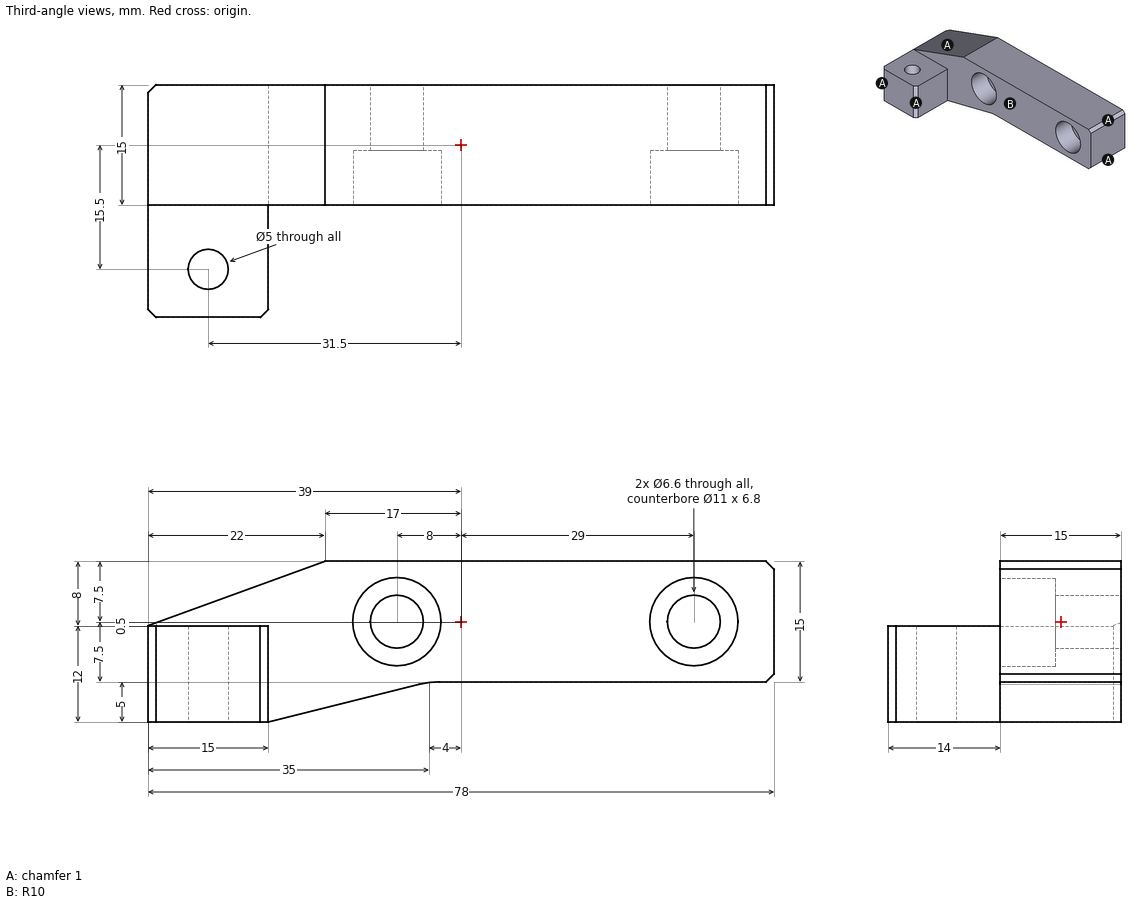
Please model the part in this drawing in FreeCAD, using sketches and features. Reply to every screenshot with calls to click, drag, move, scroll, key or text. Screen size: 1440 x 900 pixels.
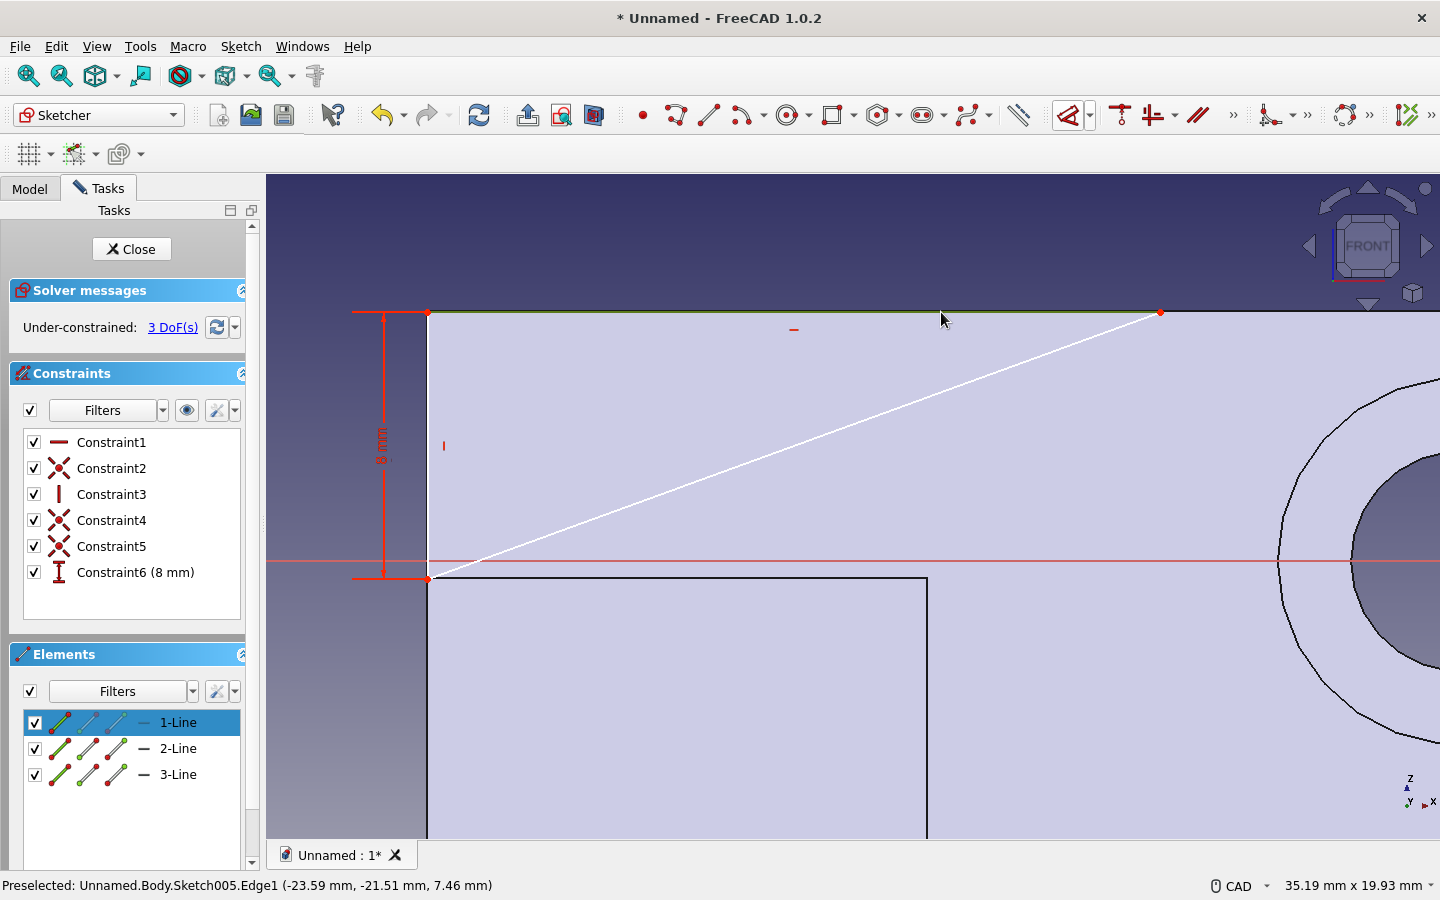
key(l)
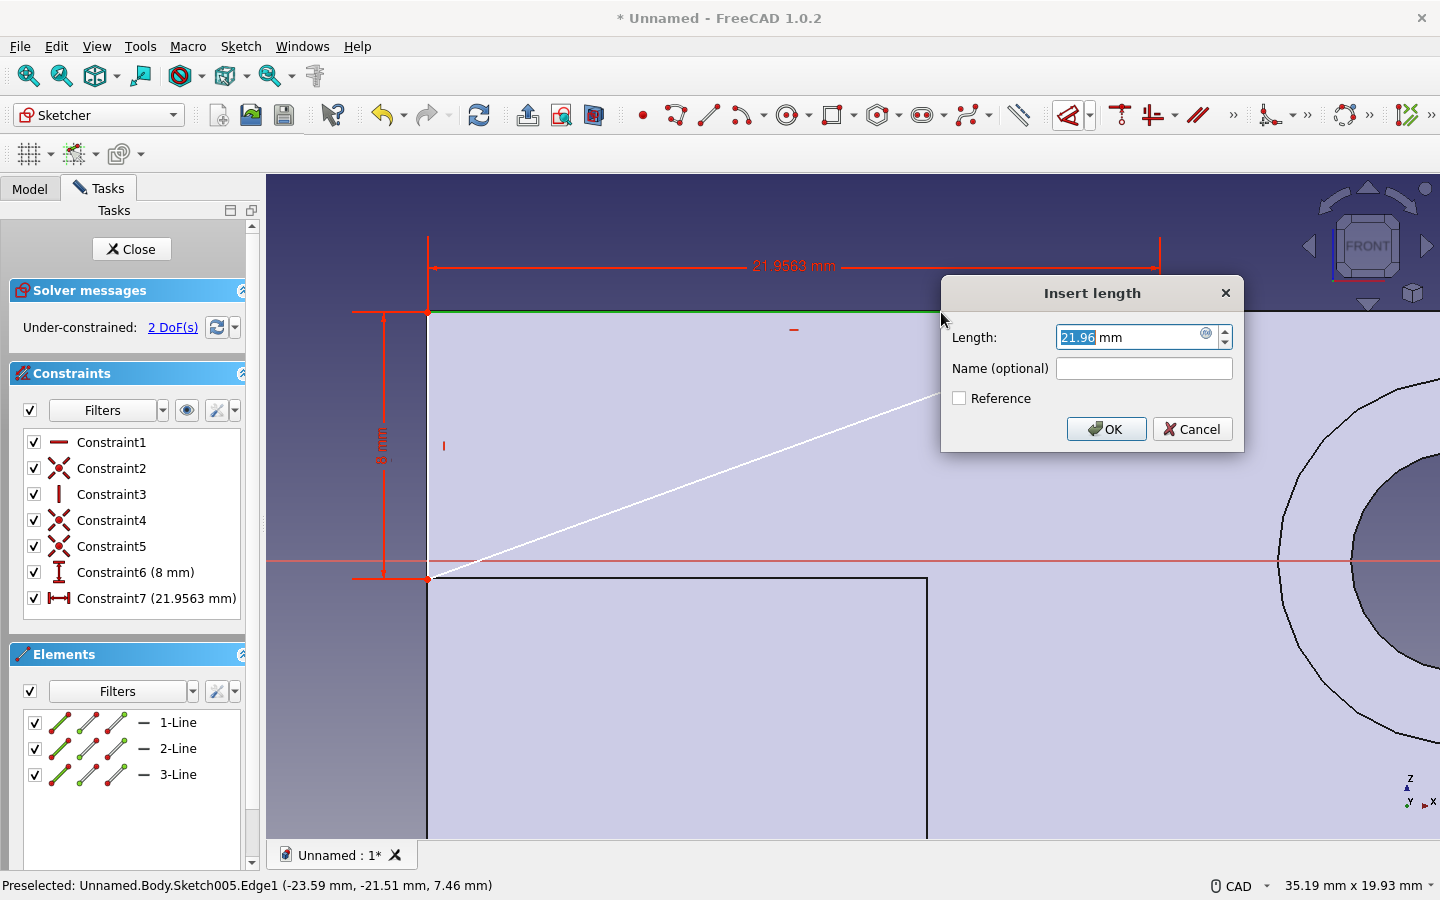
text(22)
key(Return)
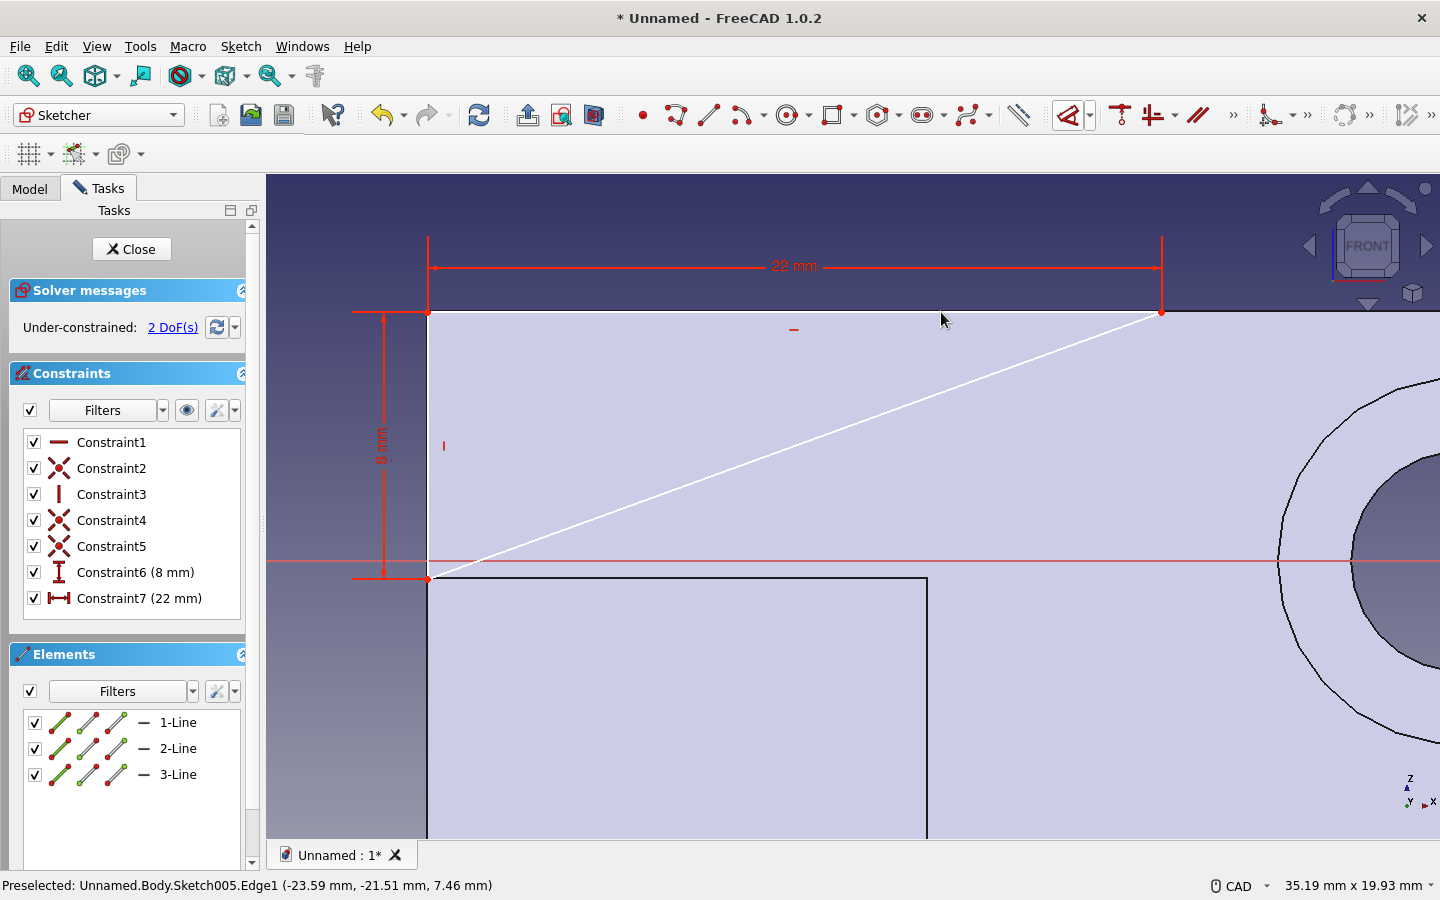
click(1162, 312)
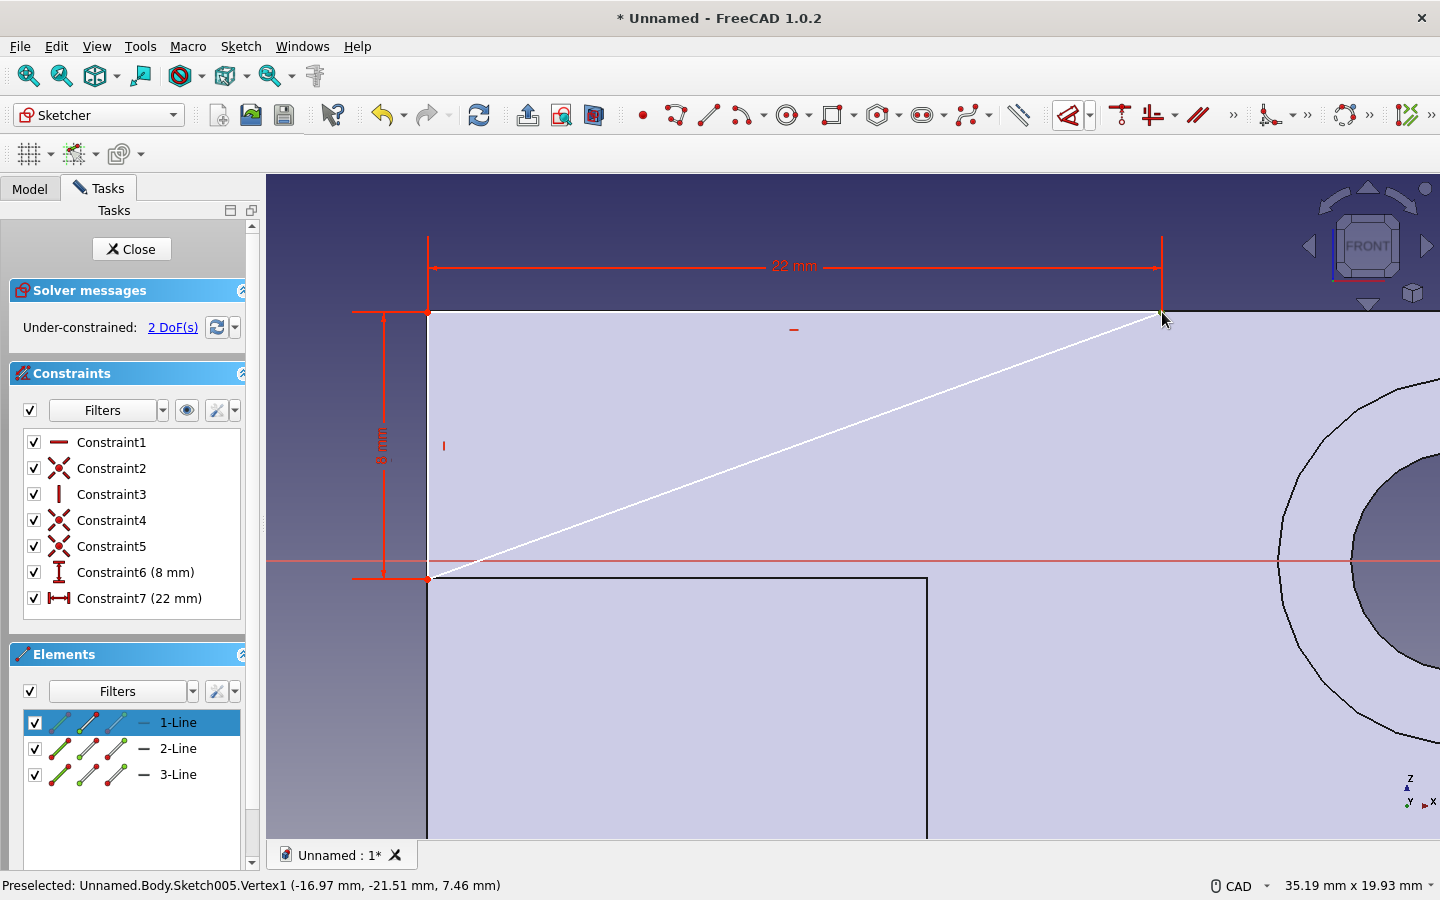
key(l)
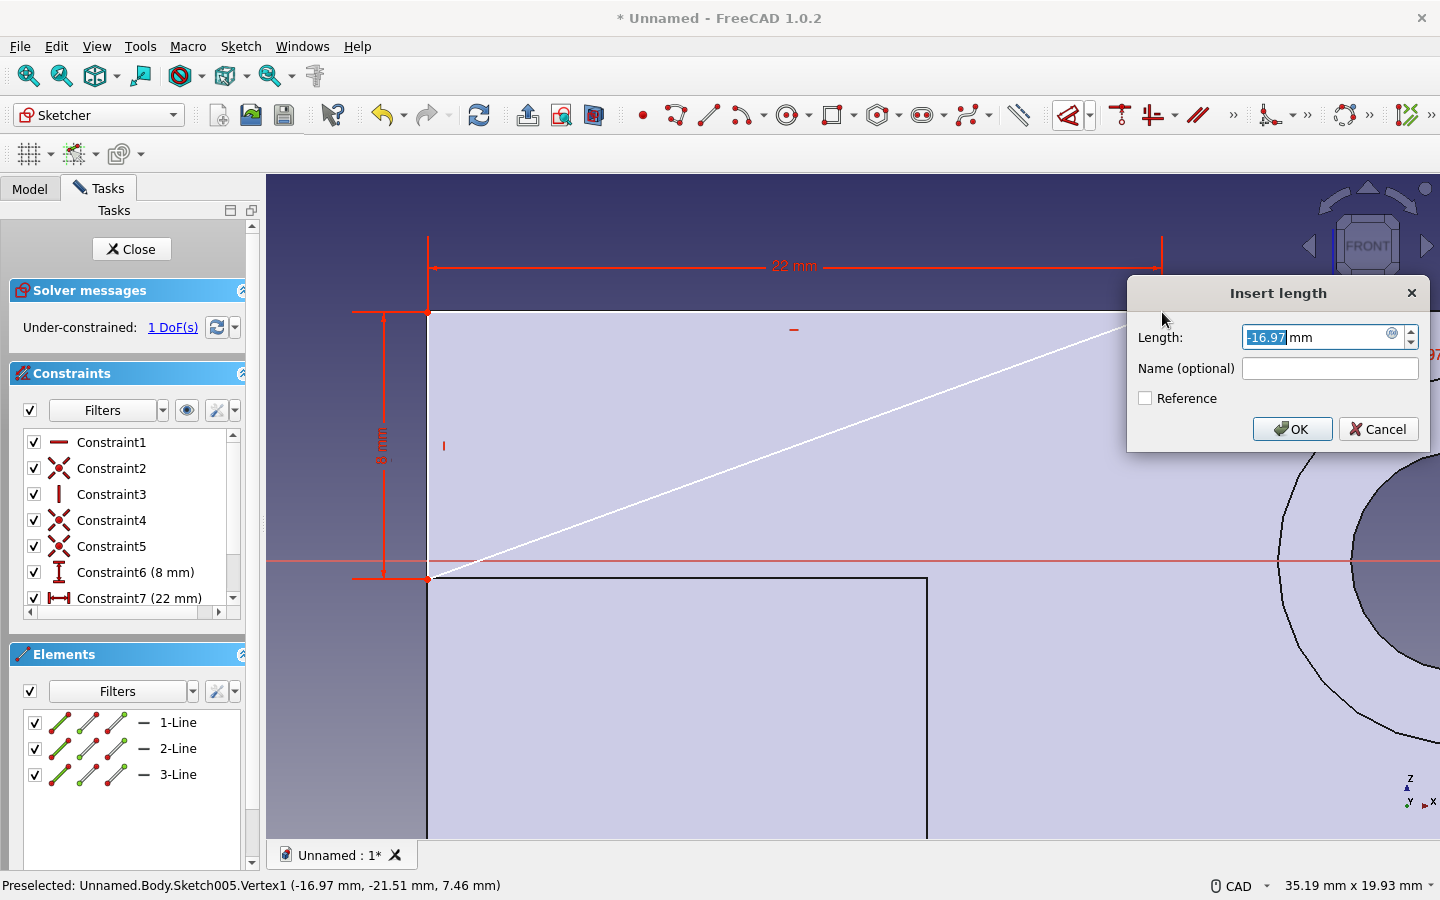
text(-17)
key(Return)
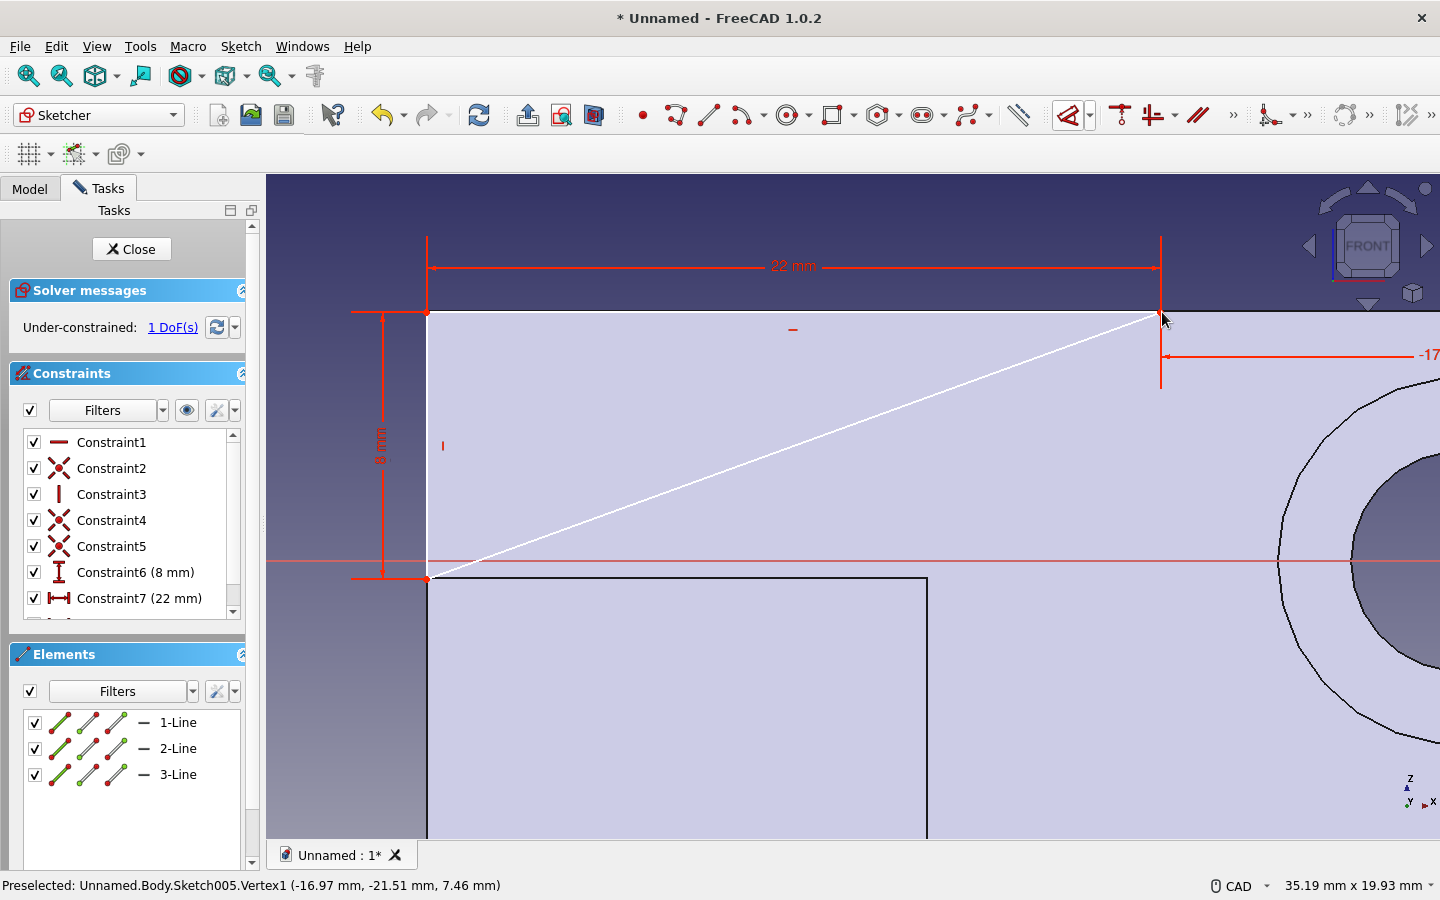
click(1161, 312)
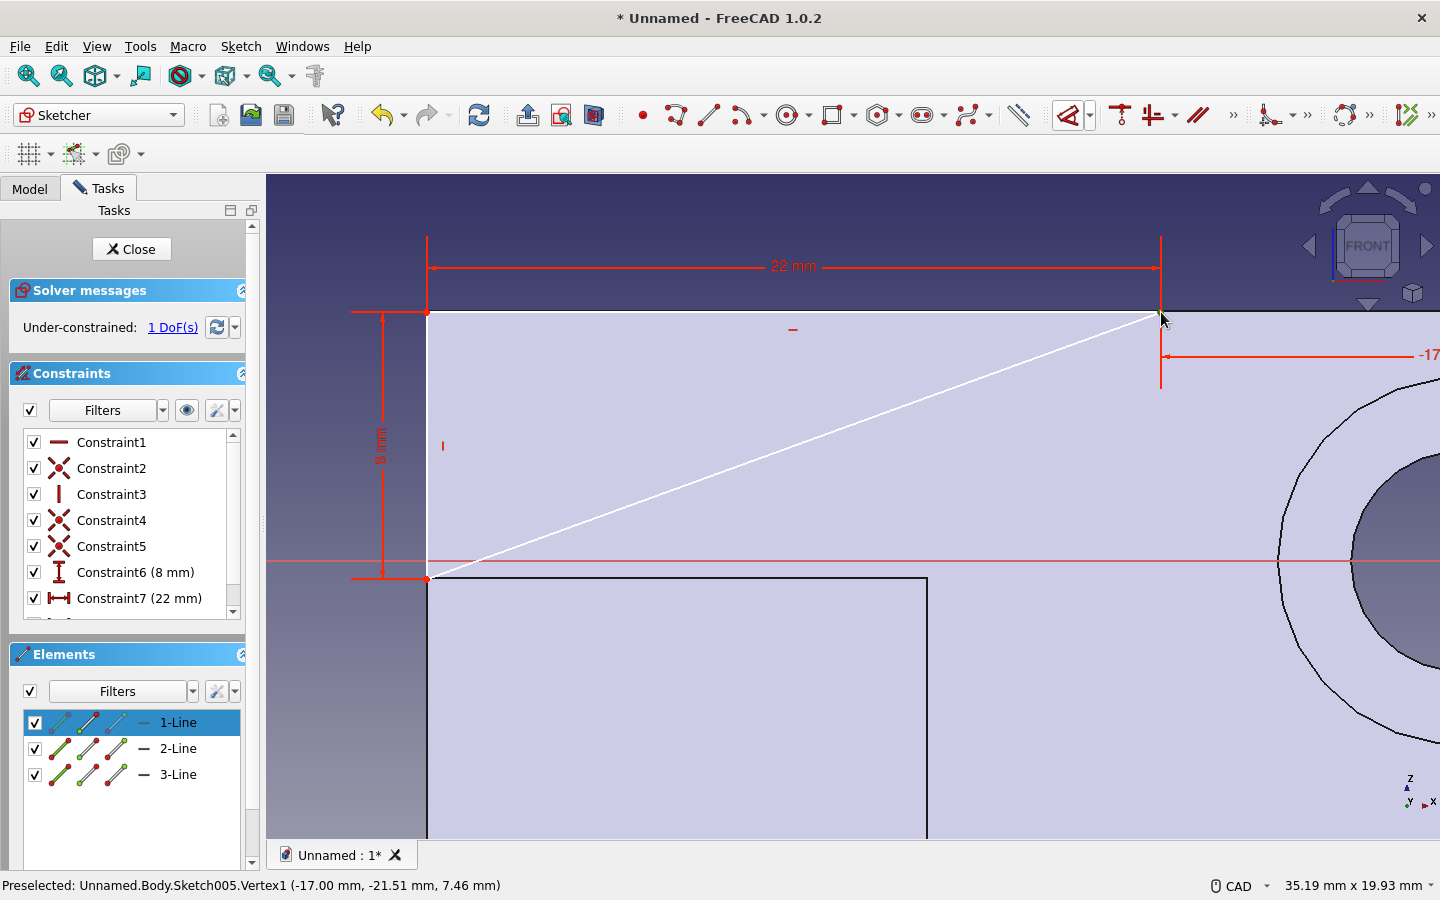
click(1090, 116)